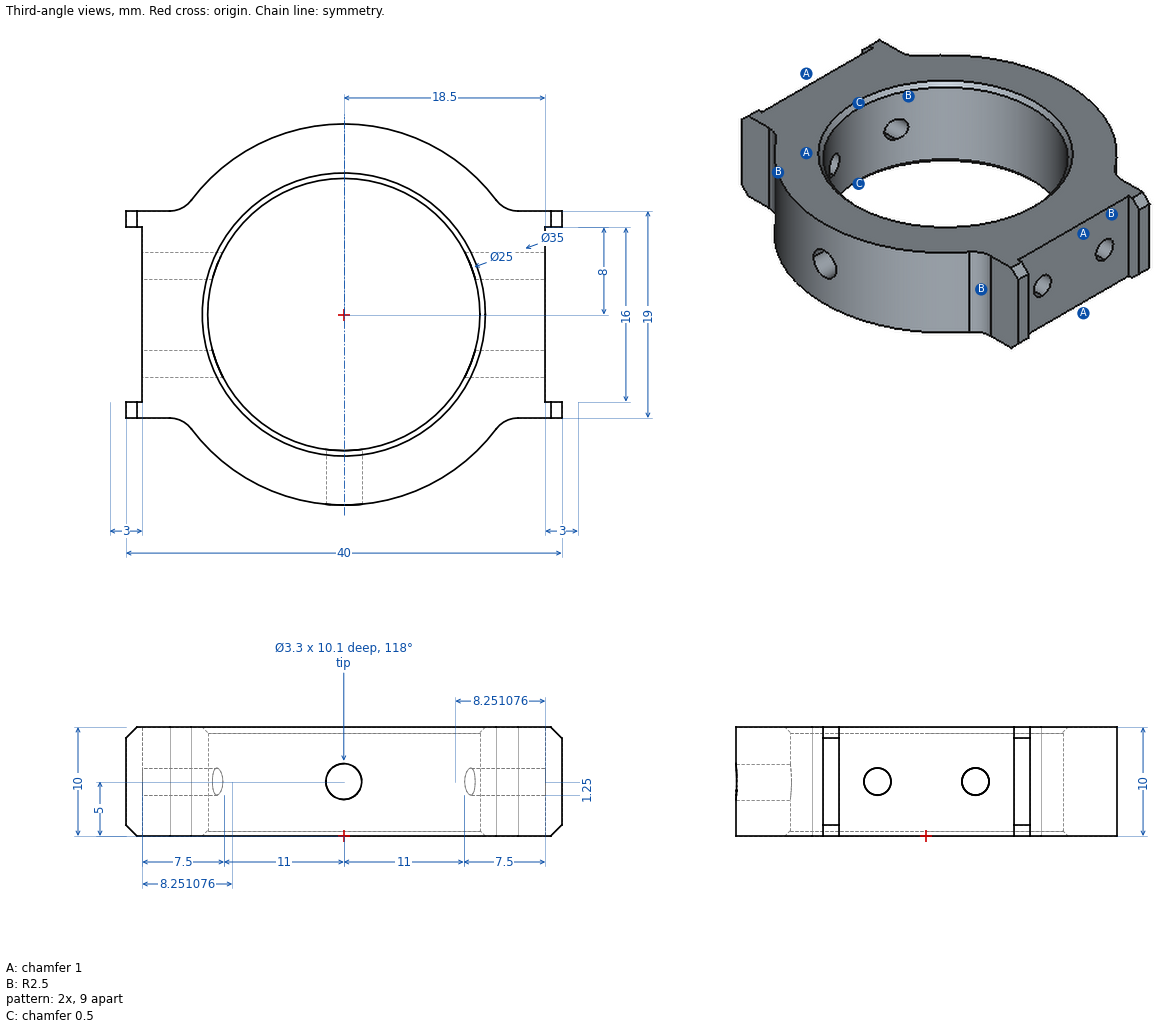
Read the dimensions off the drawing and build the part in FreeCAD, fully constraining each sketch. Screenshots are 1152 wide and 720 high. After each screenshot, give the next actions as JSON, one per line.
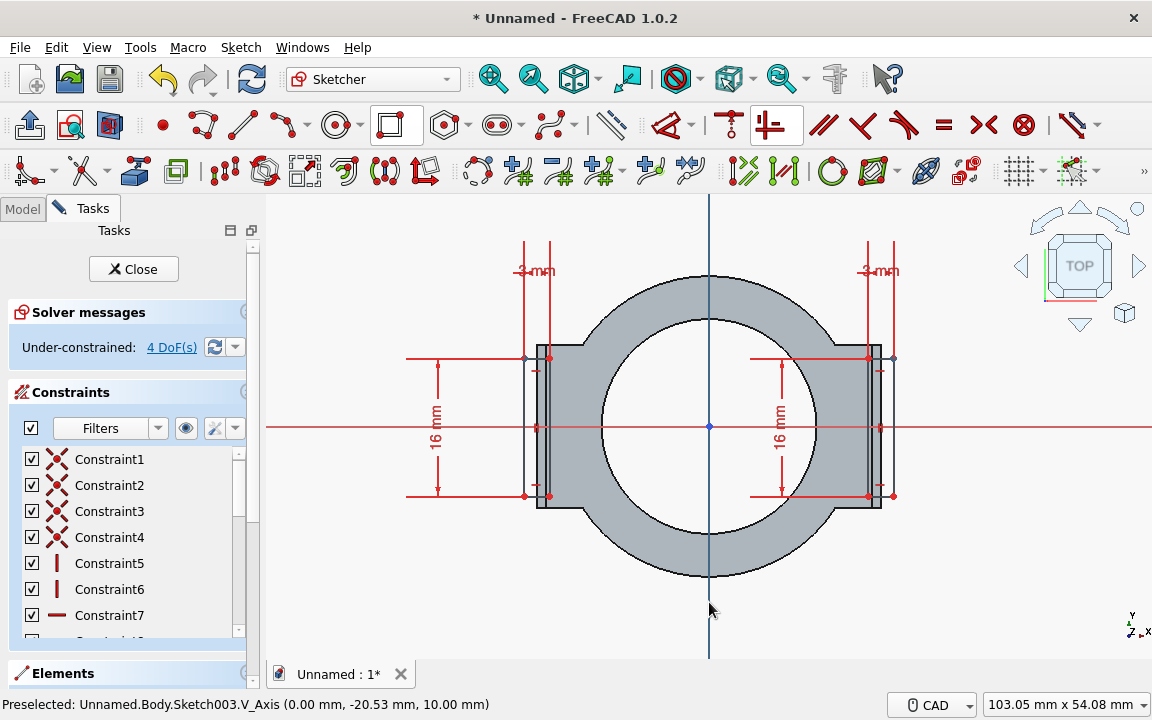
{"action": "left_click", "coordinate": [984, 126]}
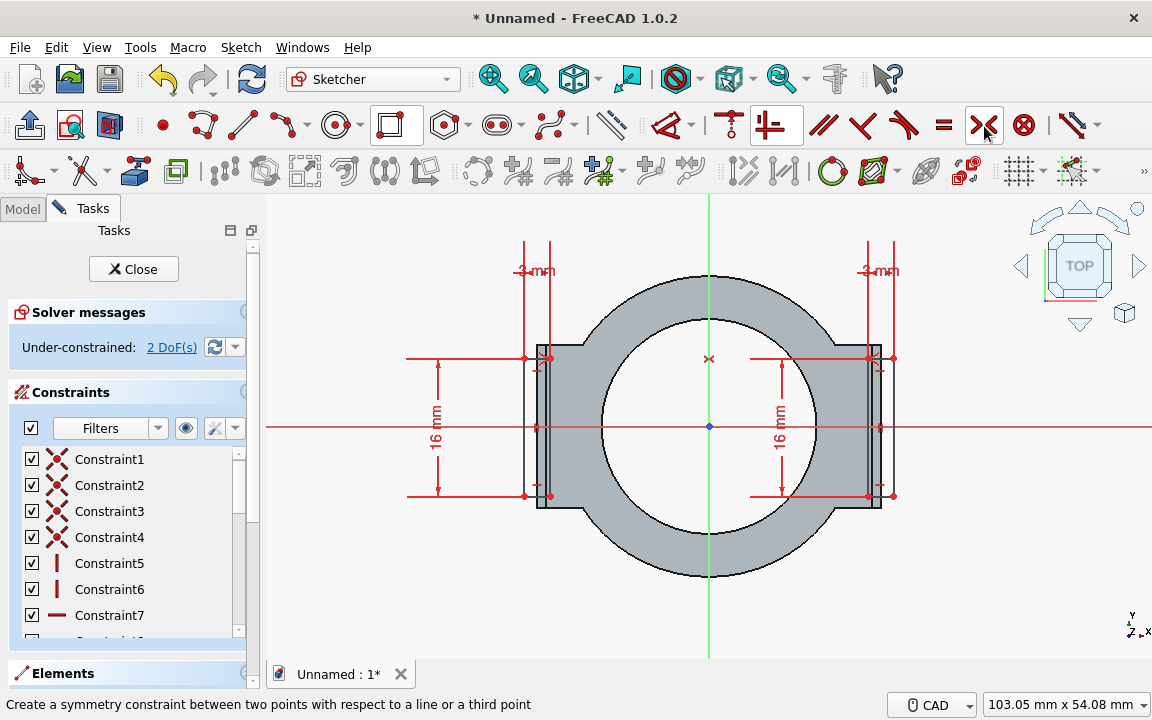
{"action": "left_click", "coordinate": [868, 359]}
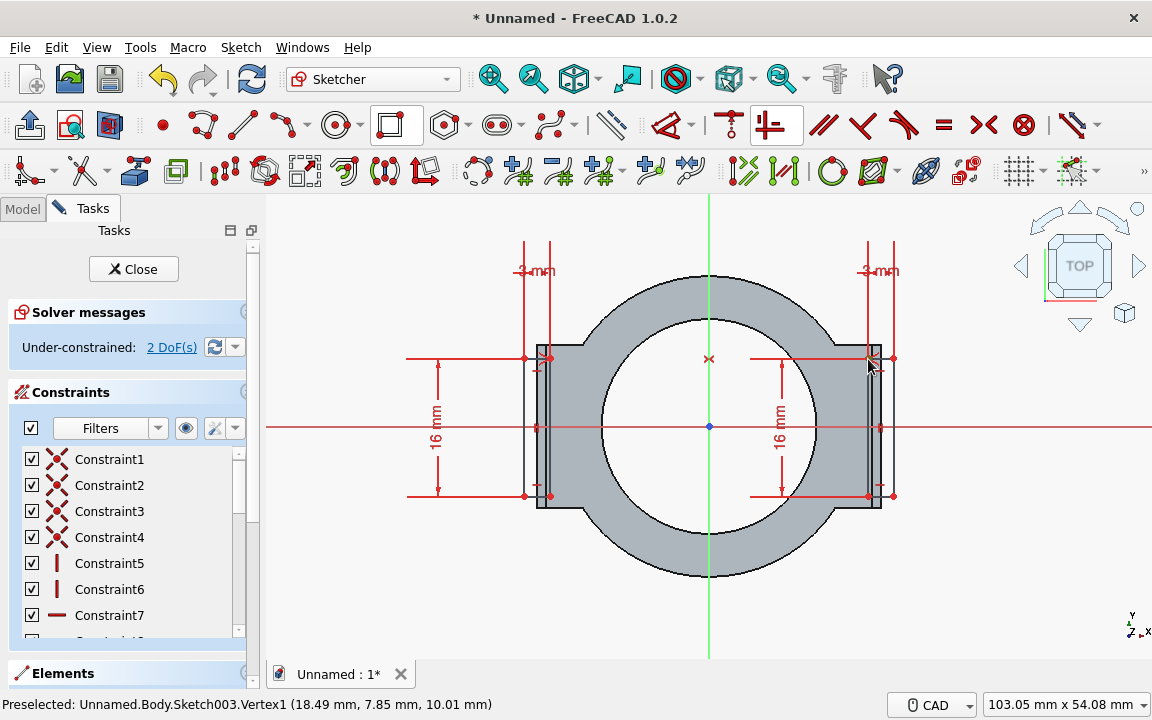
{"action": "key", "text": "i"}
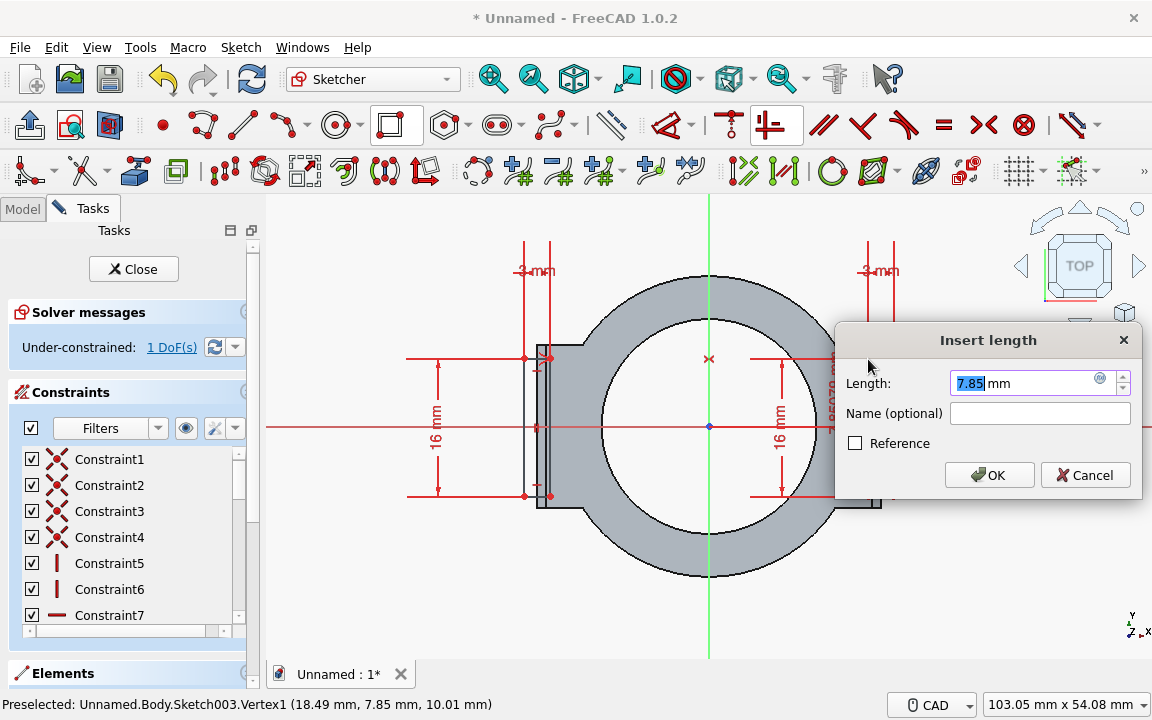
{"action": "type", "text": "8"}
{"action": "key", "text": "Return"}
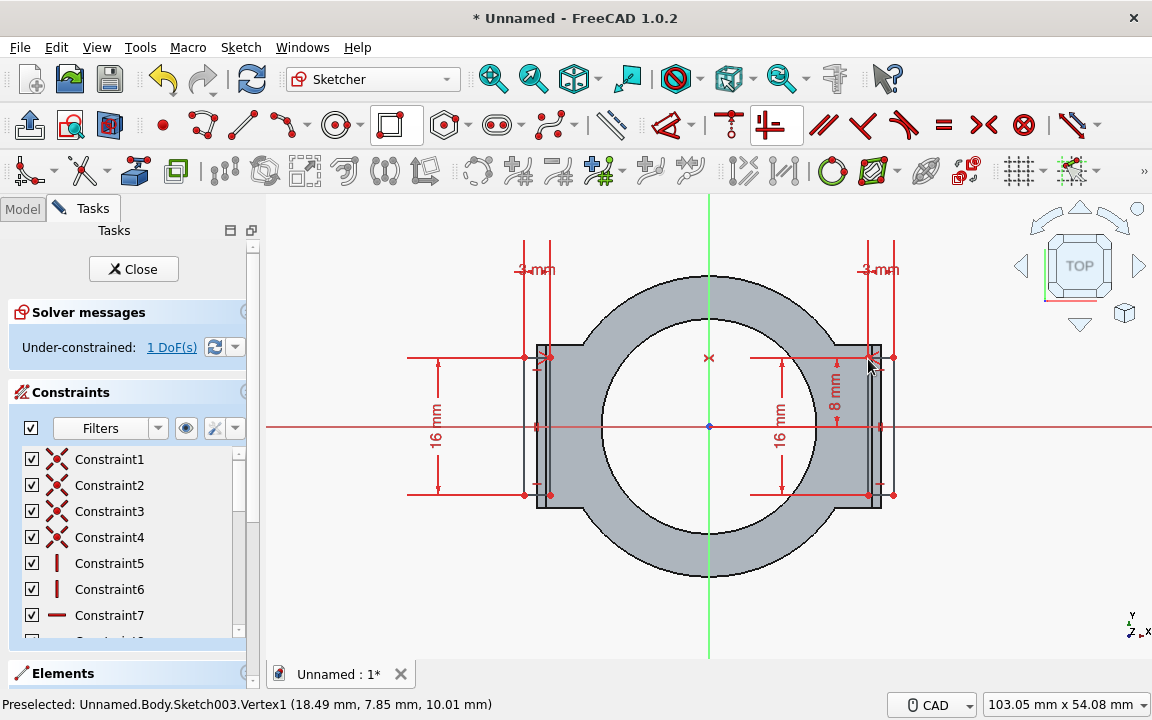
{"action": "left_click", "coordinate": [868, 358]}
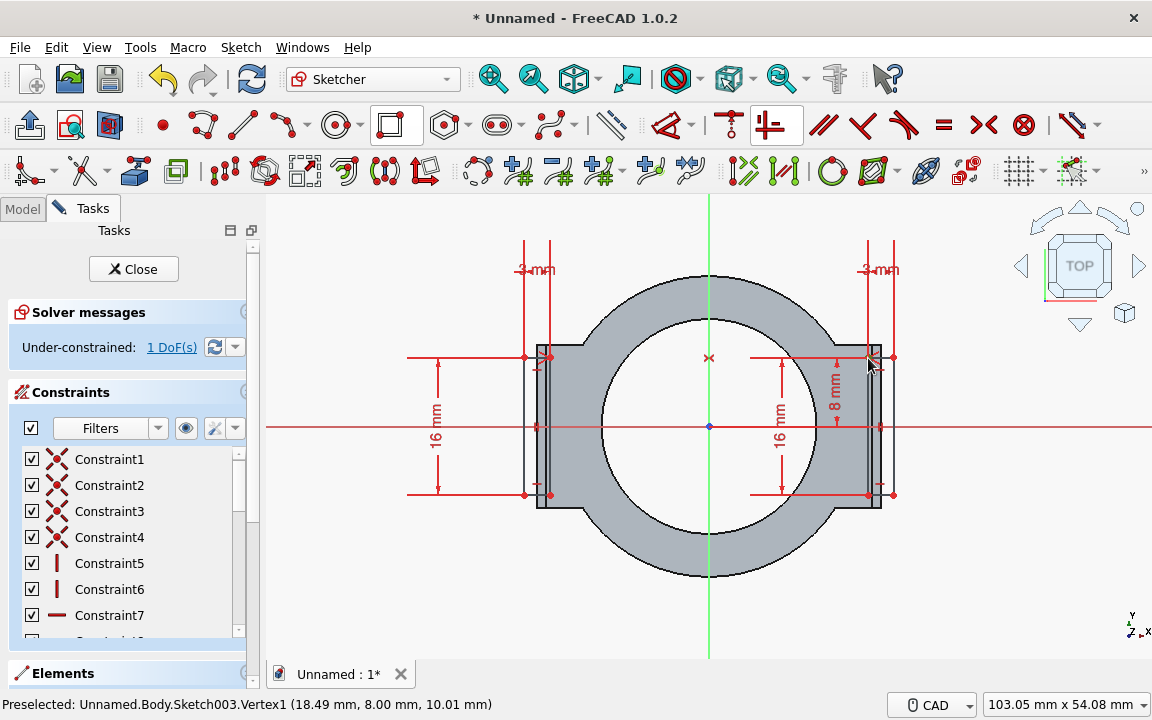
{"action": "left_click", "coordinate": [694, 126]}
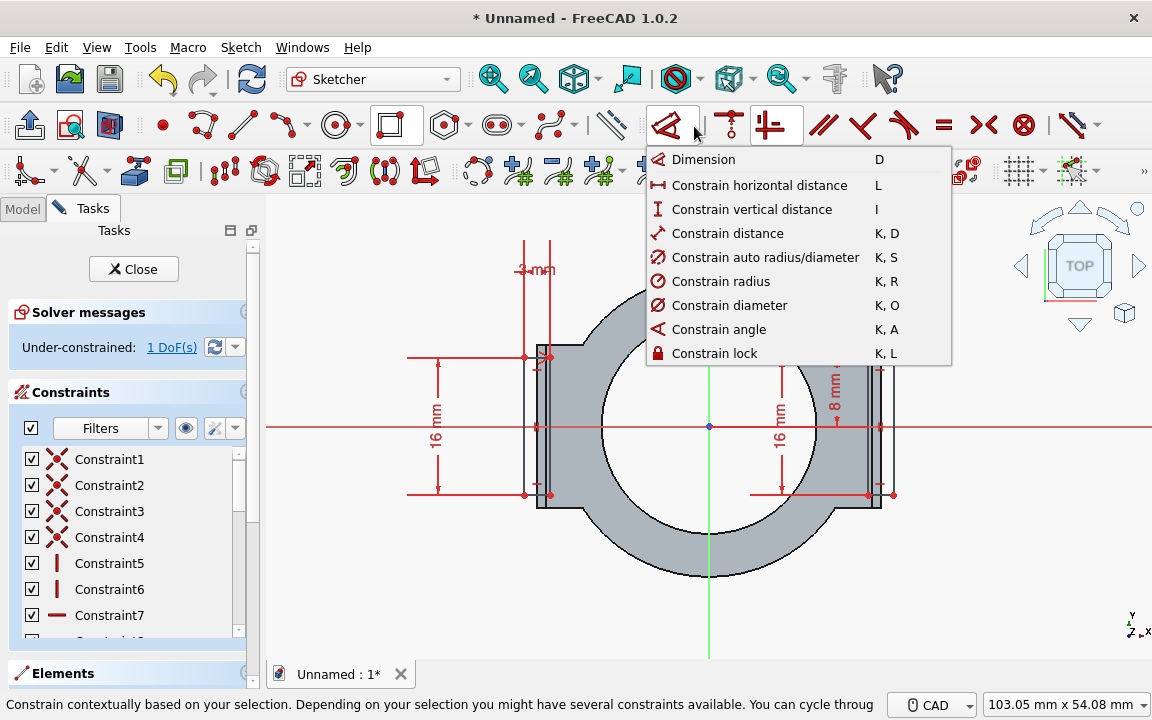
{"action": "left_click", "coordinate": [799, 185]}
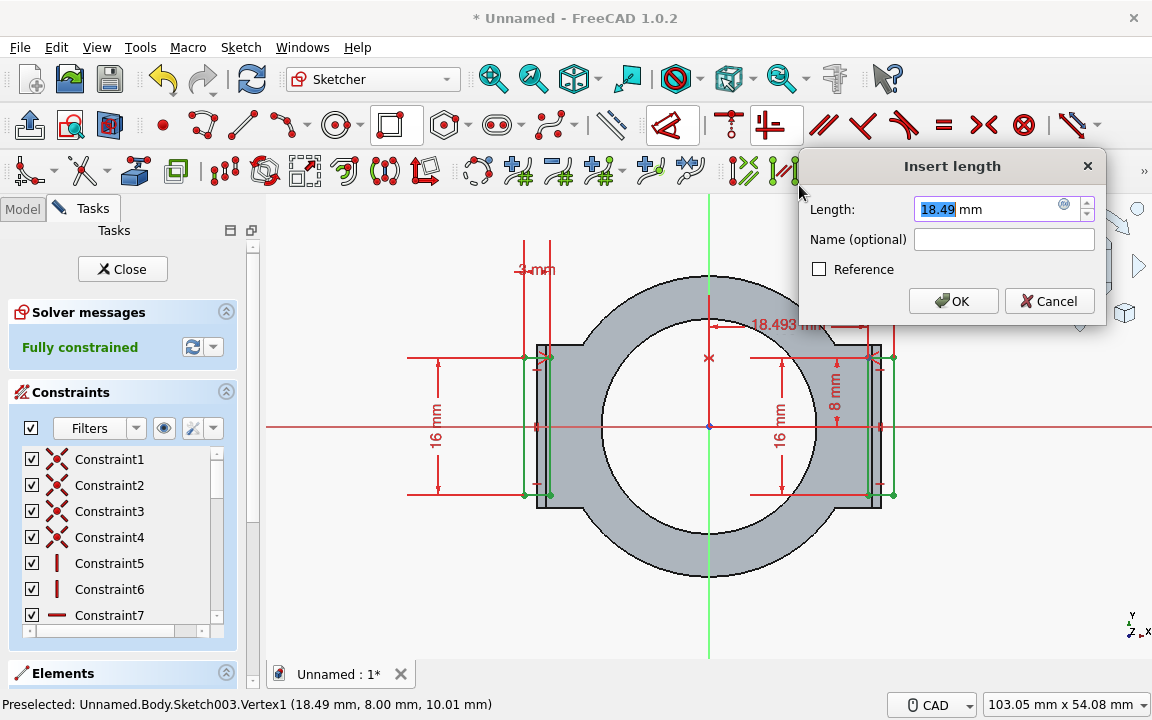
{"action": "type", "text": "18.5"}
{"action": "key", "text": "Return"}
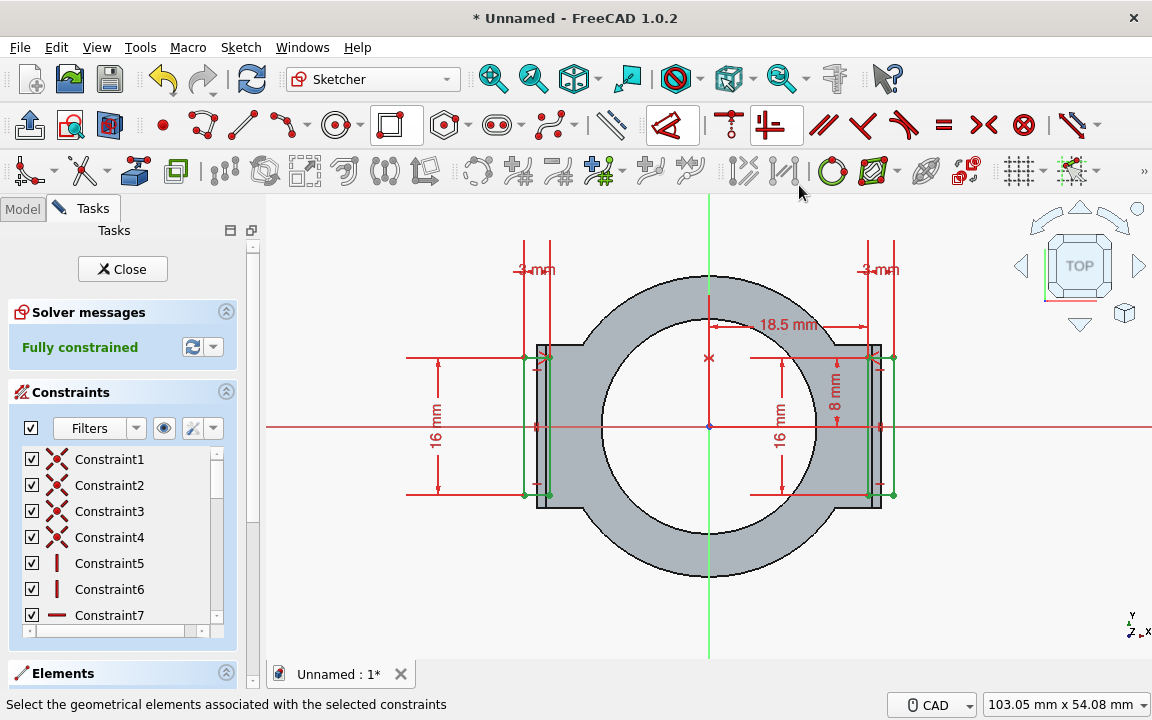
{"action": "left_click", "coordinate": [123, 269]}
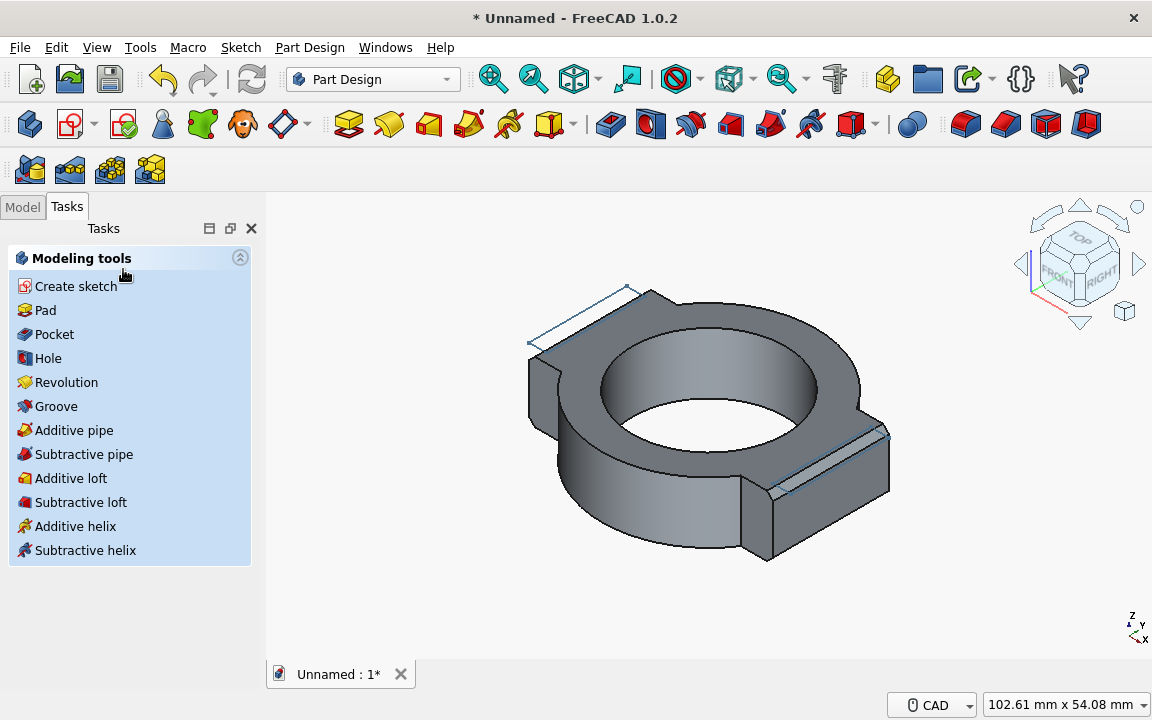
{"action": "left_click", "coordinate": [612, 124]}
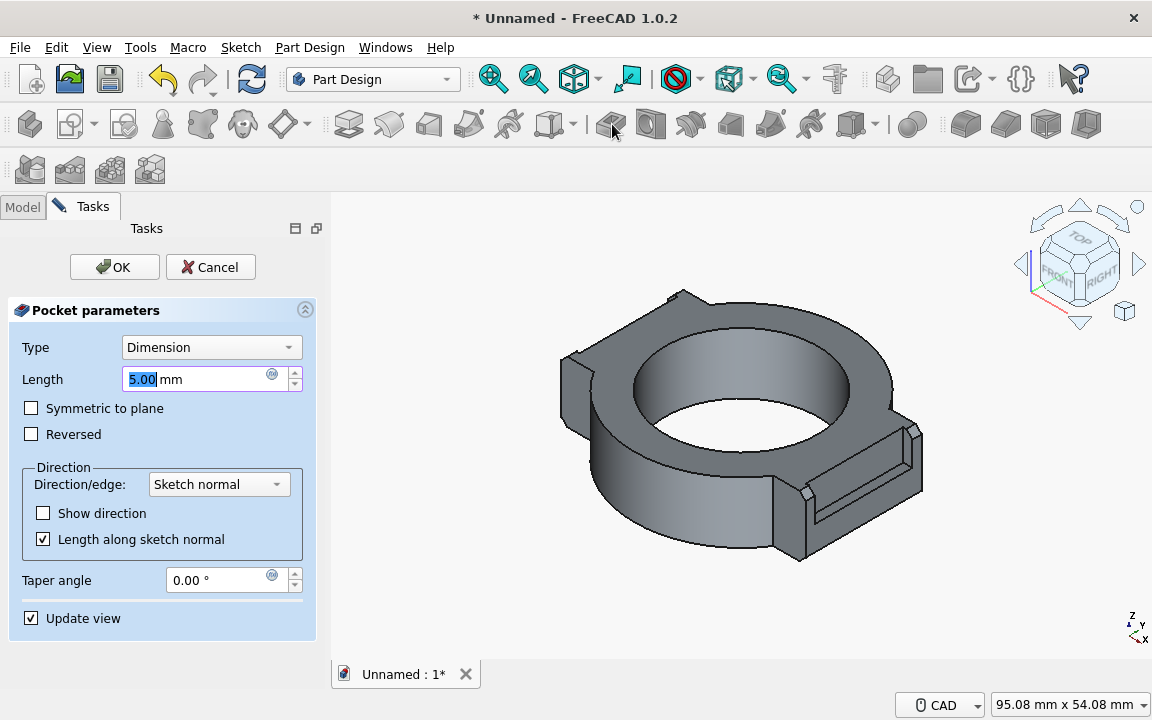
{"action": "left_click", "coordinate": [212, 348]}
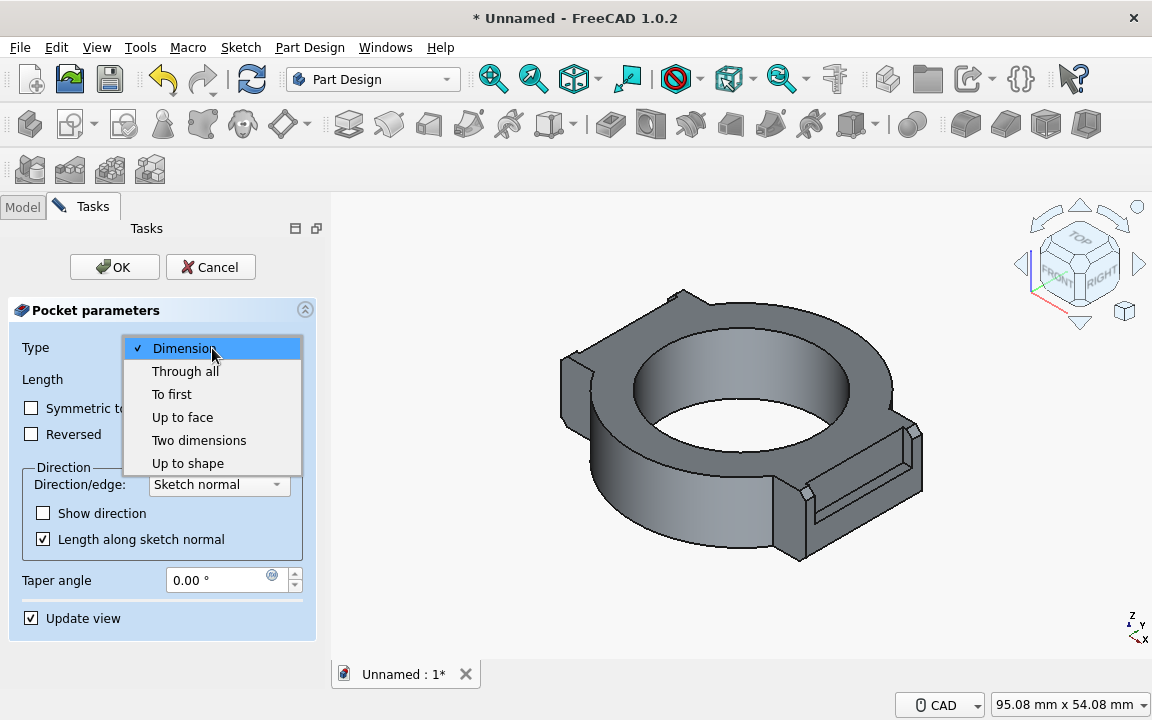
{"action": "left_click", "coordinate": [212, 372]}